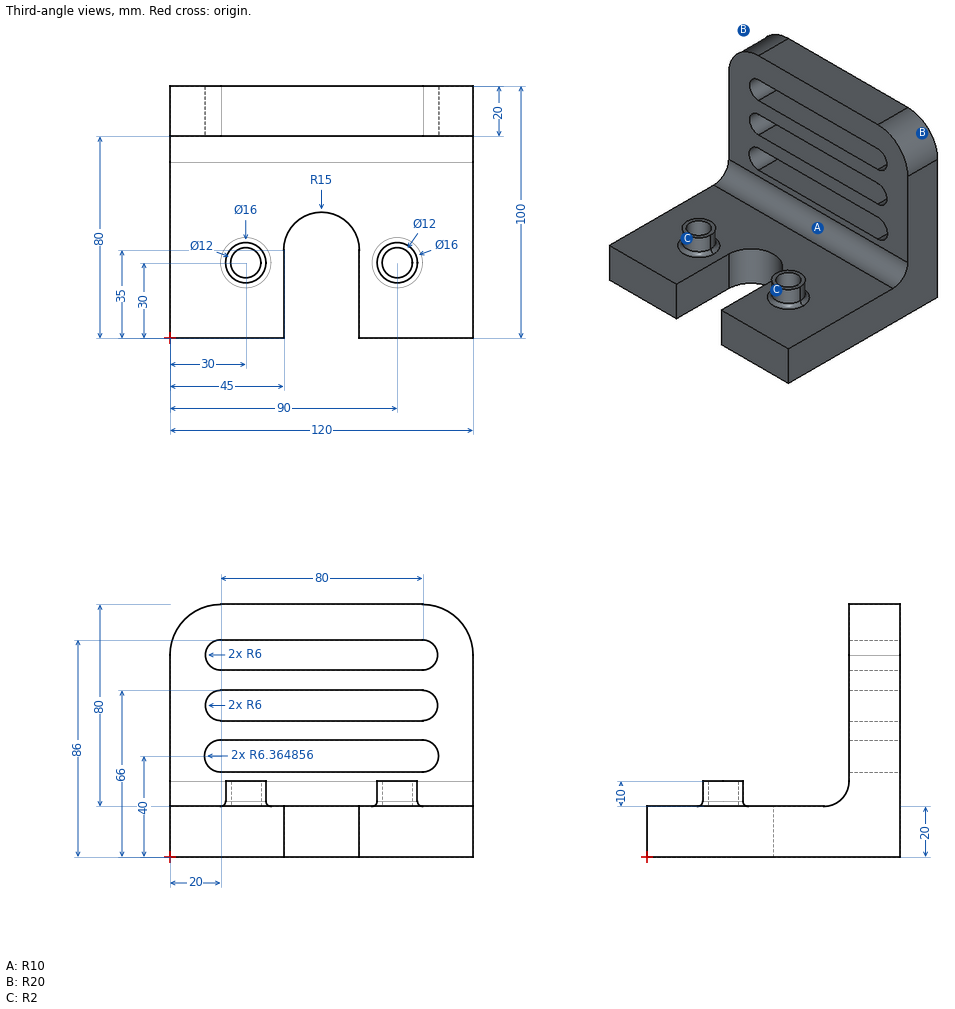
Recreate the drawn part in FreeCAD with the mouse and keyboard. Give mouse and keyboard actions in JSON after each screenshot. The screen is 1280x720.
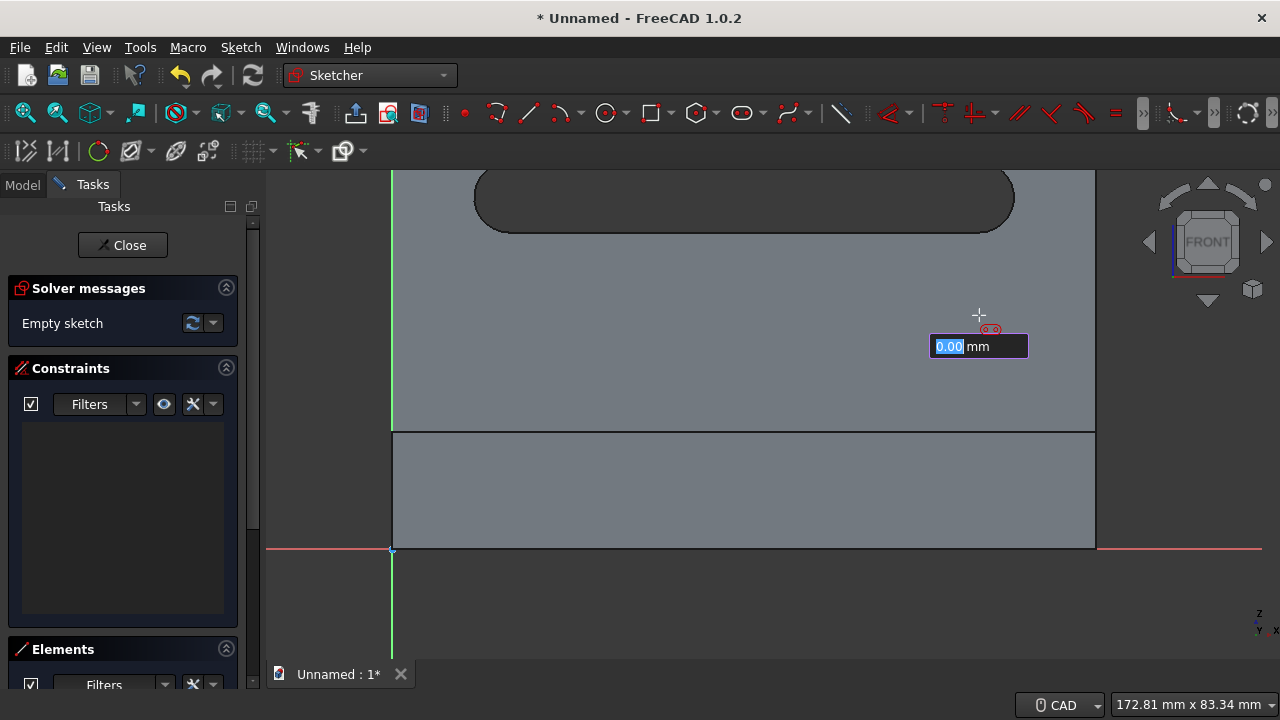
{"action": "left_click", "coordinate": [744, 277]}
{"action": "key", "text": "Escape"}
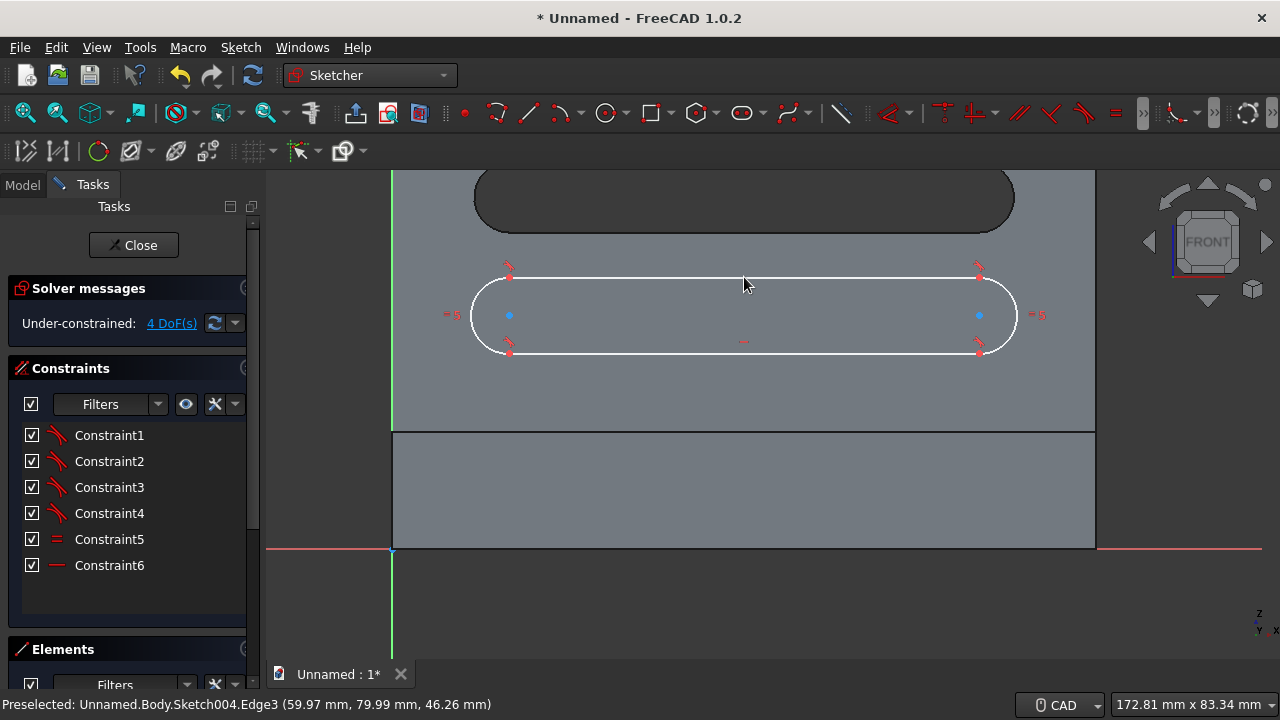
{"action": "key", "text": "d"}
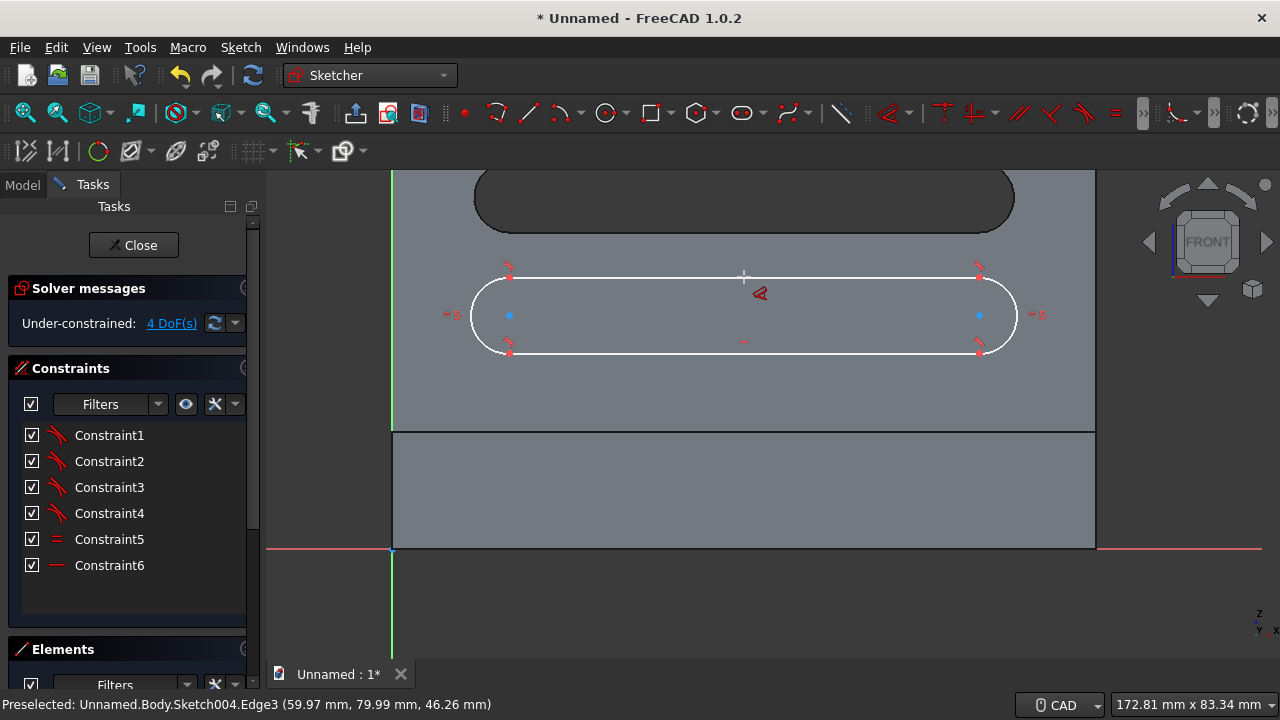
{"action": "left_click", "coordinate": [478, 294]}
{"action": "left_click", "coordinate": [452, 275]}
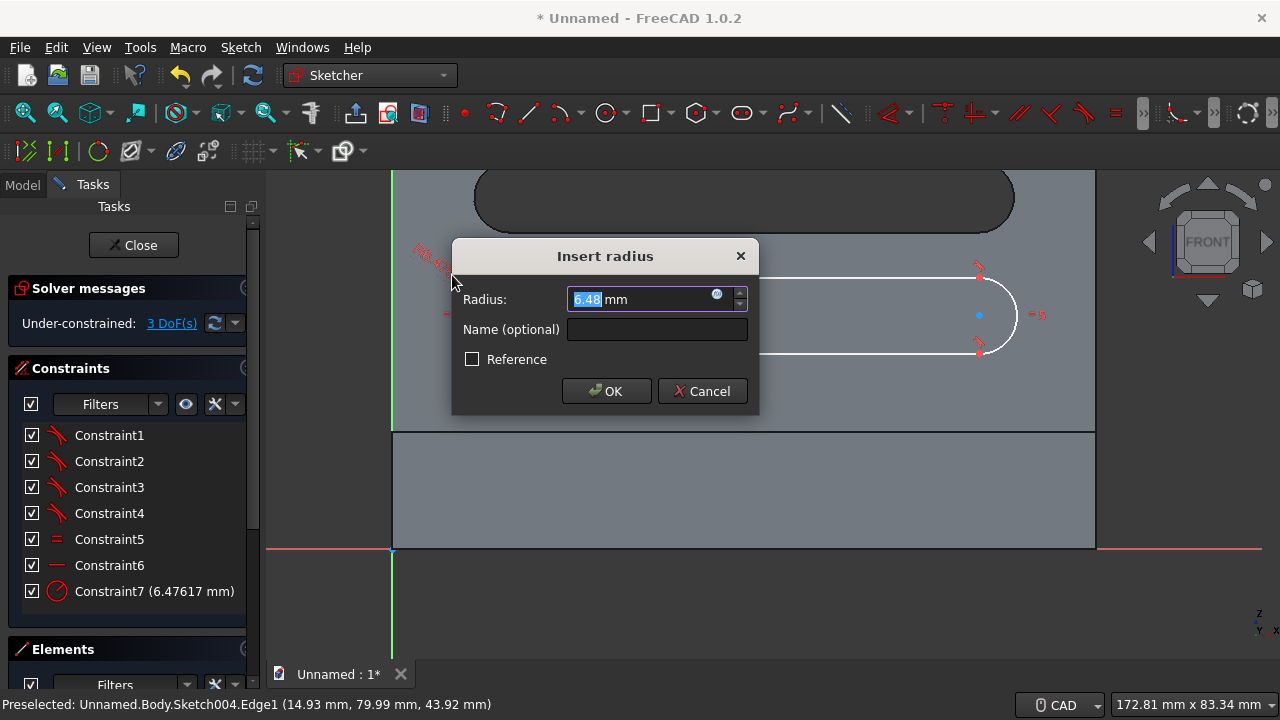
{"action": "type", "text": "6.364856"}
{"action": "key", "text": "Return"}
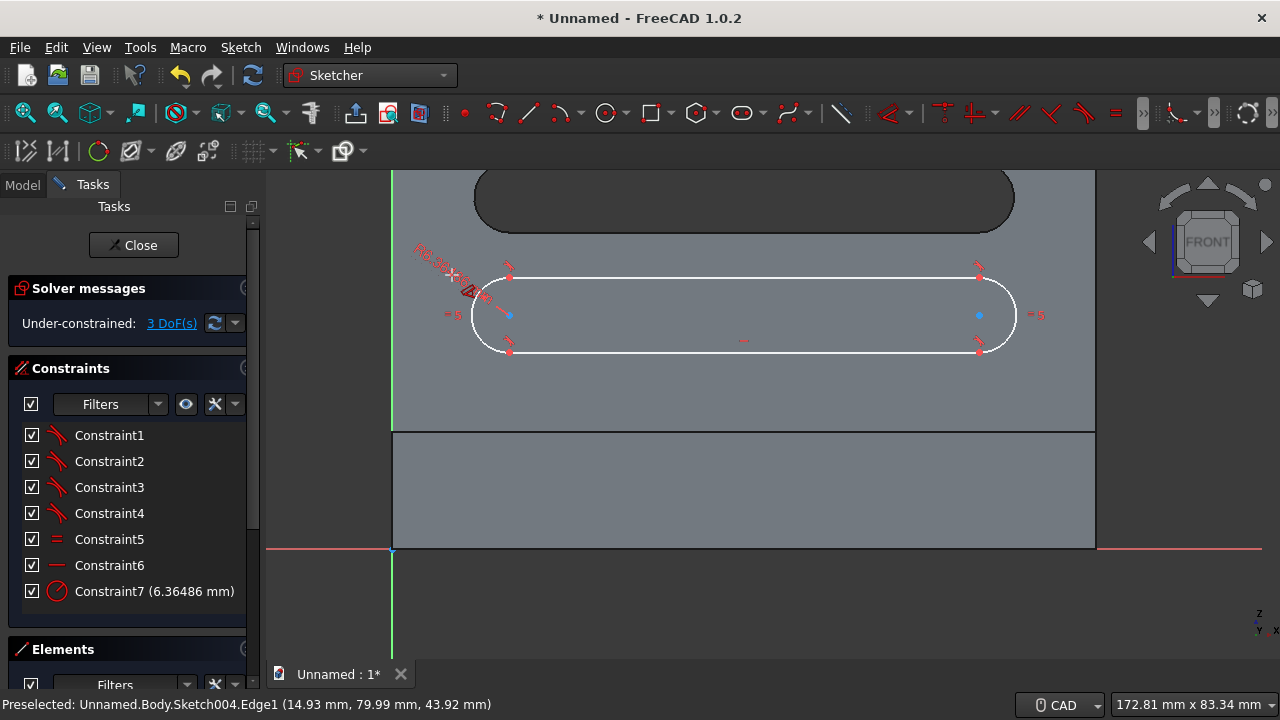
{"action": "left_click", "coordinate": [650, 278]}
{"action": "left_click", "coordinate": [744, 244]}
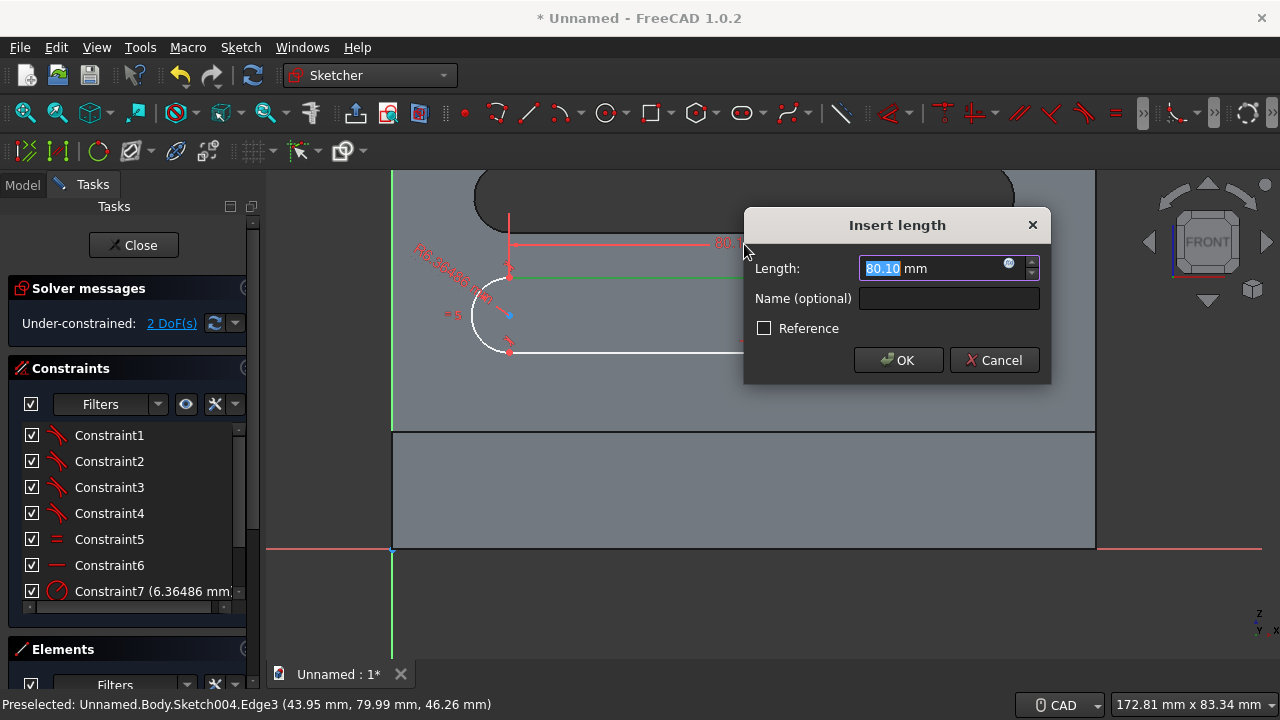
{"action": "type", "text": "80"}
{"action": "key", "text": "Return"}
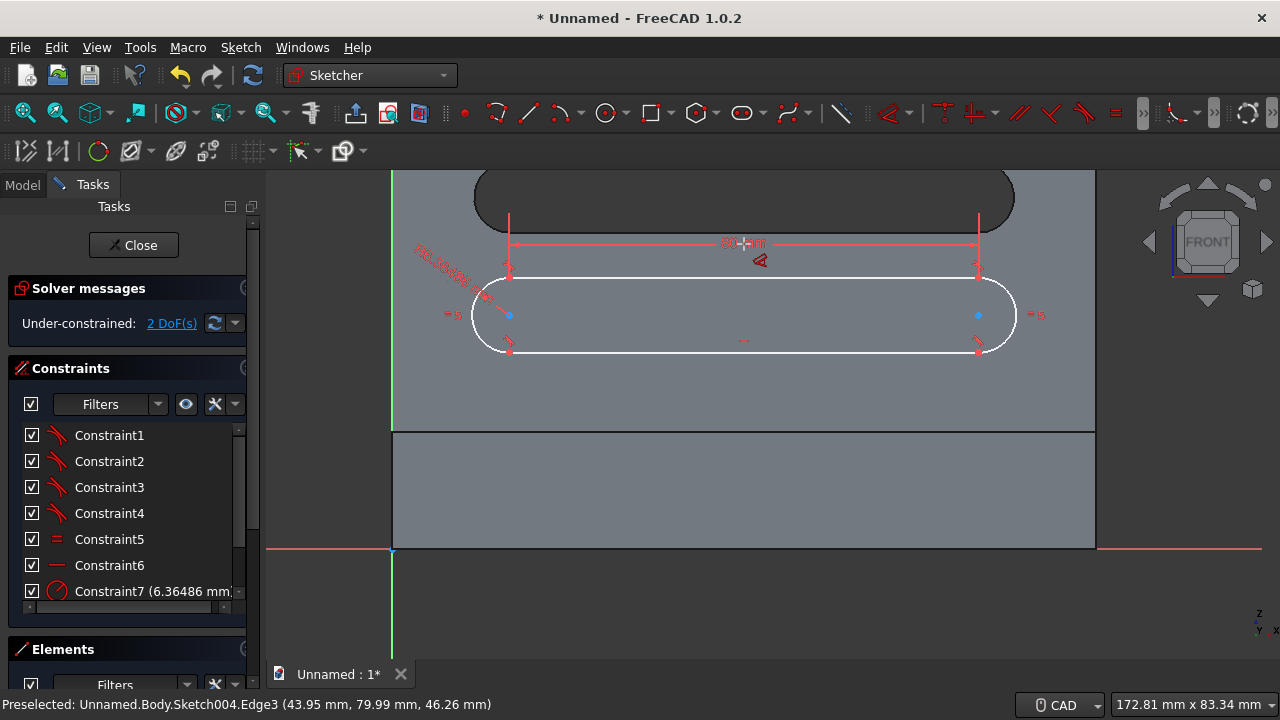
{"action": "left_click", "coordinate": [509, 278]}
{"action": "left_click", "coordinate": [451, 583]}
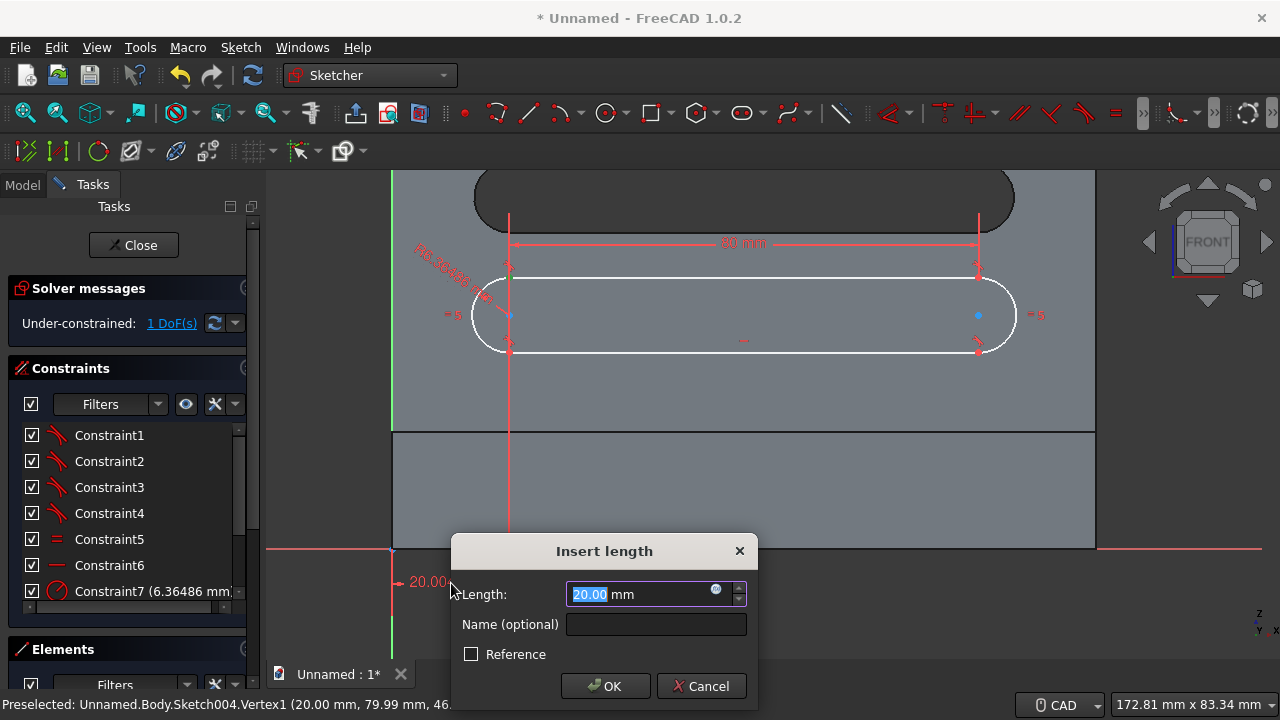
{"action": "type", "text": "20"}
{"action": "key", "text": "Return"}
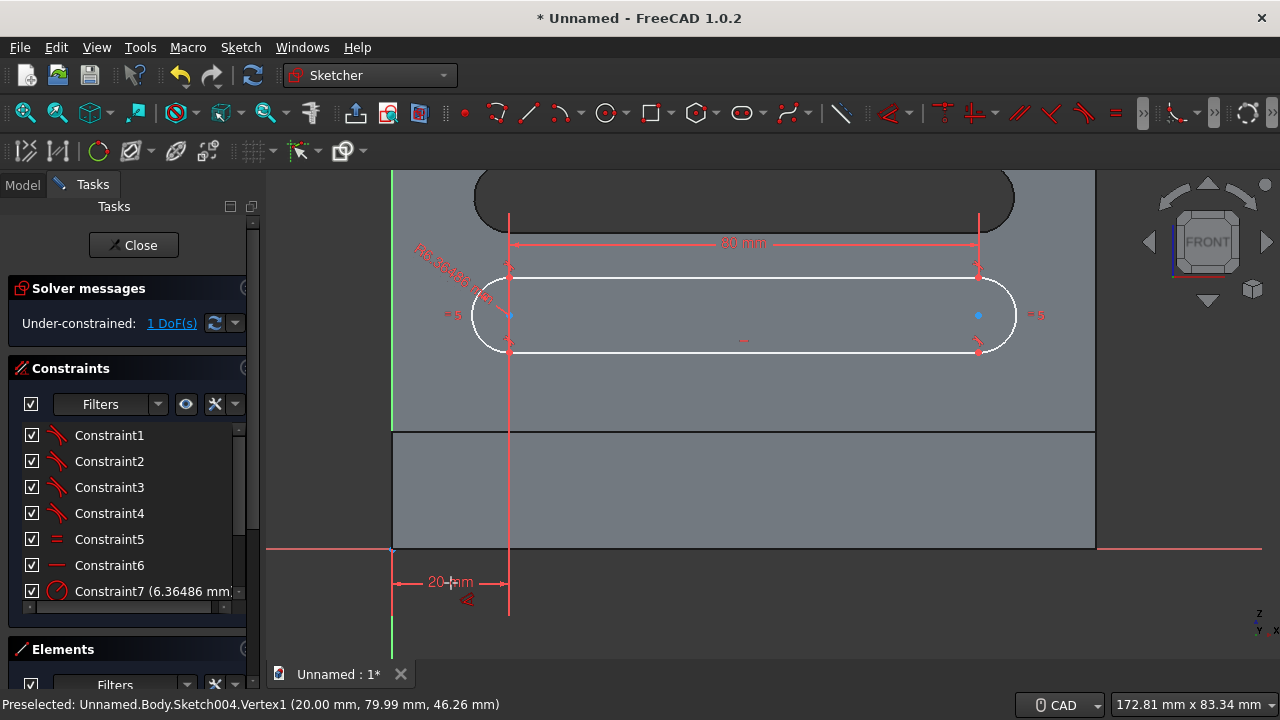
{"action": "left_click", "coordinate": [509, 315]}
{"action": "left_click", "coordinate": [358, 432]}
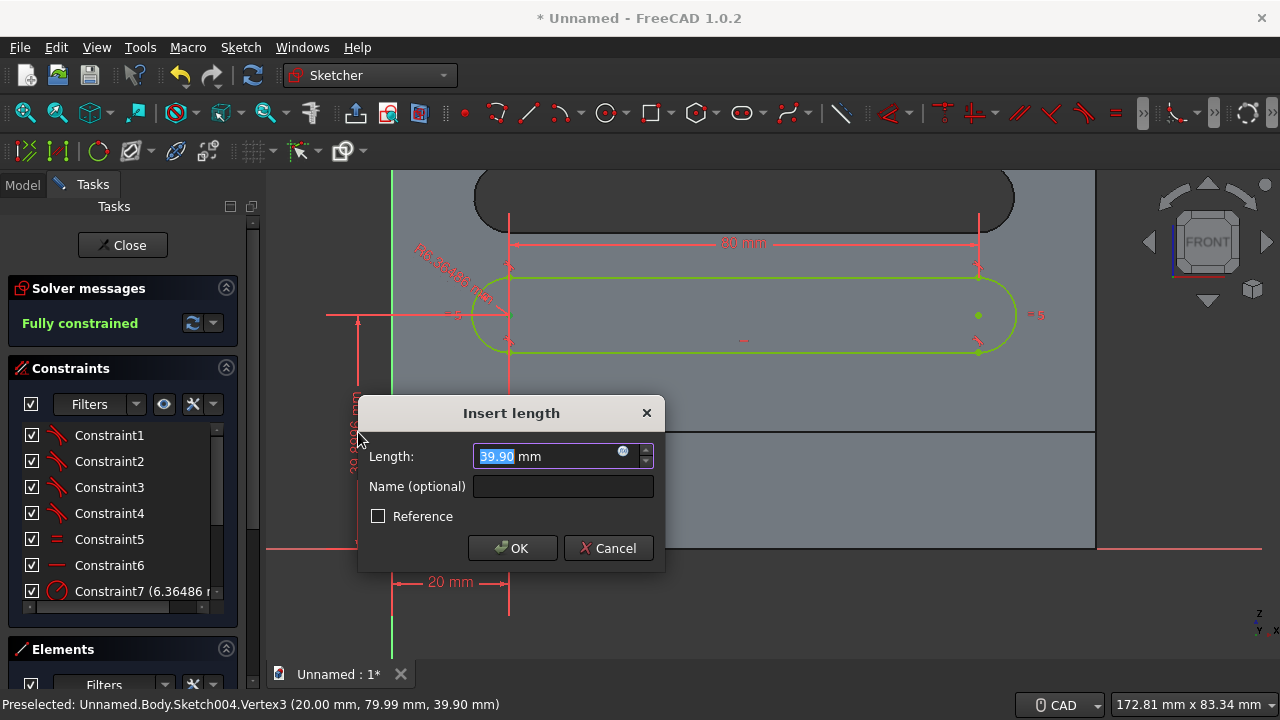
{"action": "type", "text": "40"}
{"action": "key", "text": "Return"}
{"action": "key", "text": "Escape"}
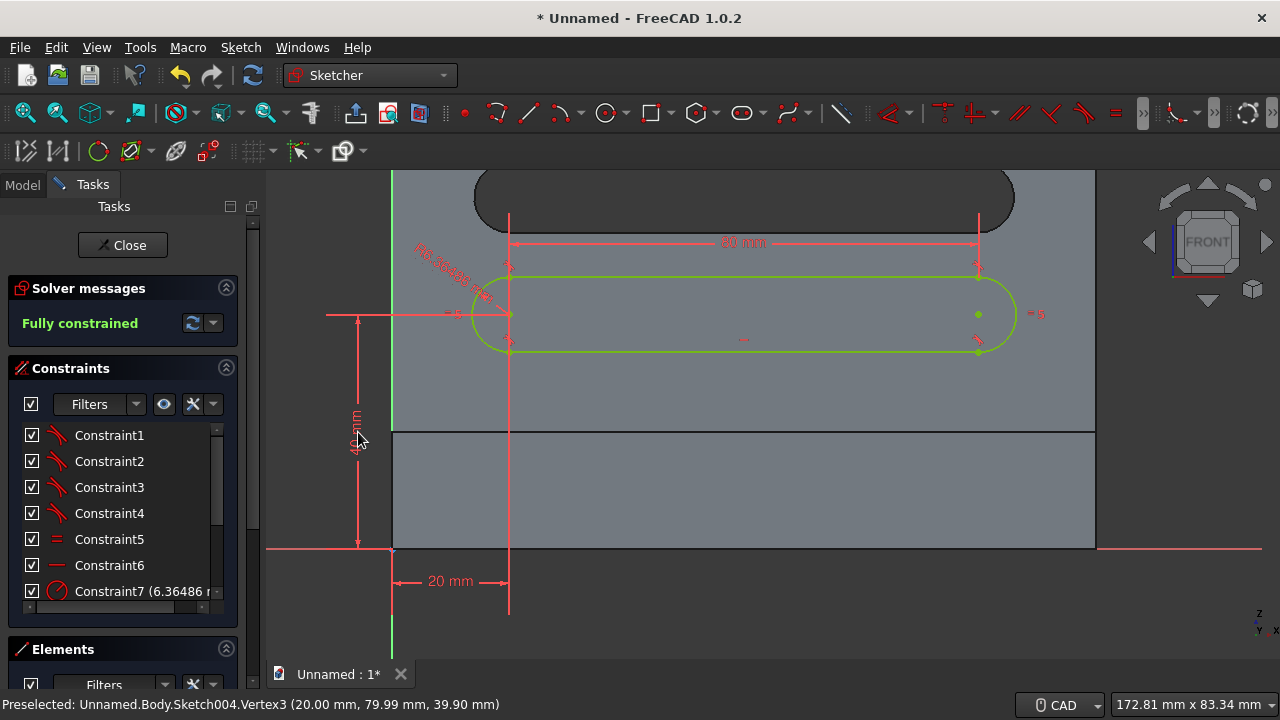
{"action": "left_click", "coordinate": [123, 245]}